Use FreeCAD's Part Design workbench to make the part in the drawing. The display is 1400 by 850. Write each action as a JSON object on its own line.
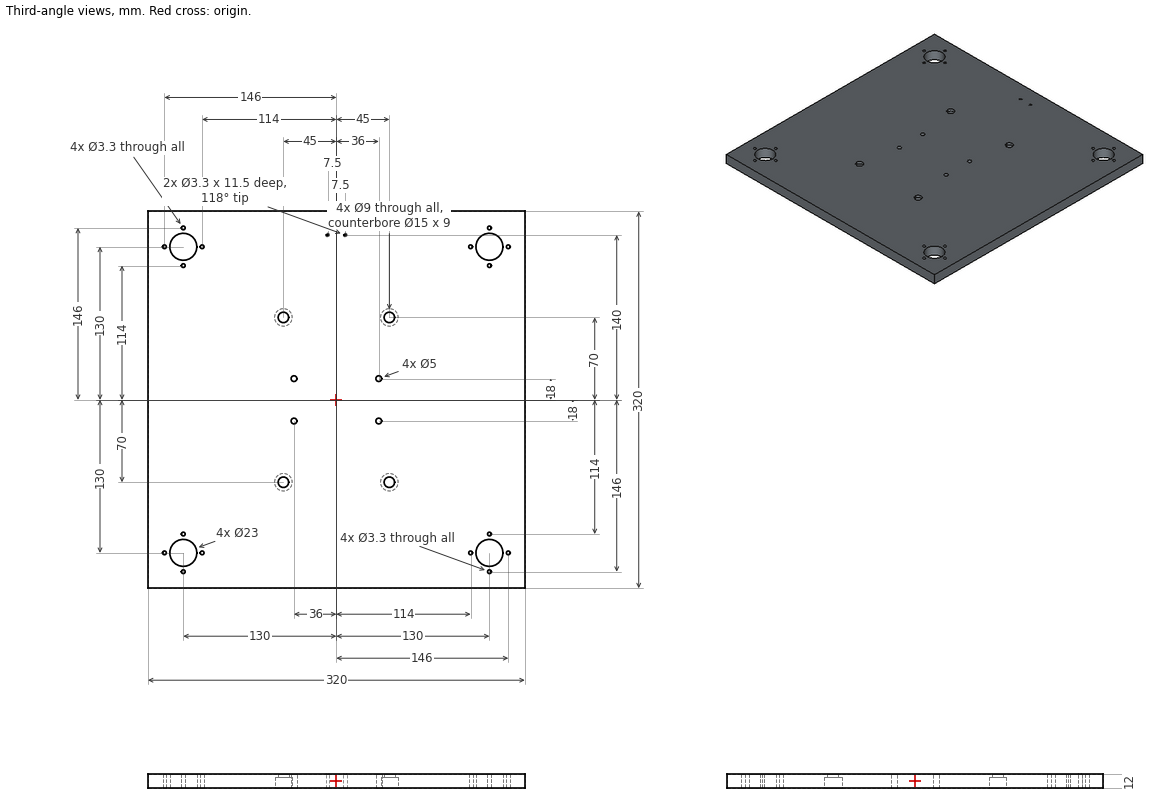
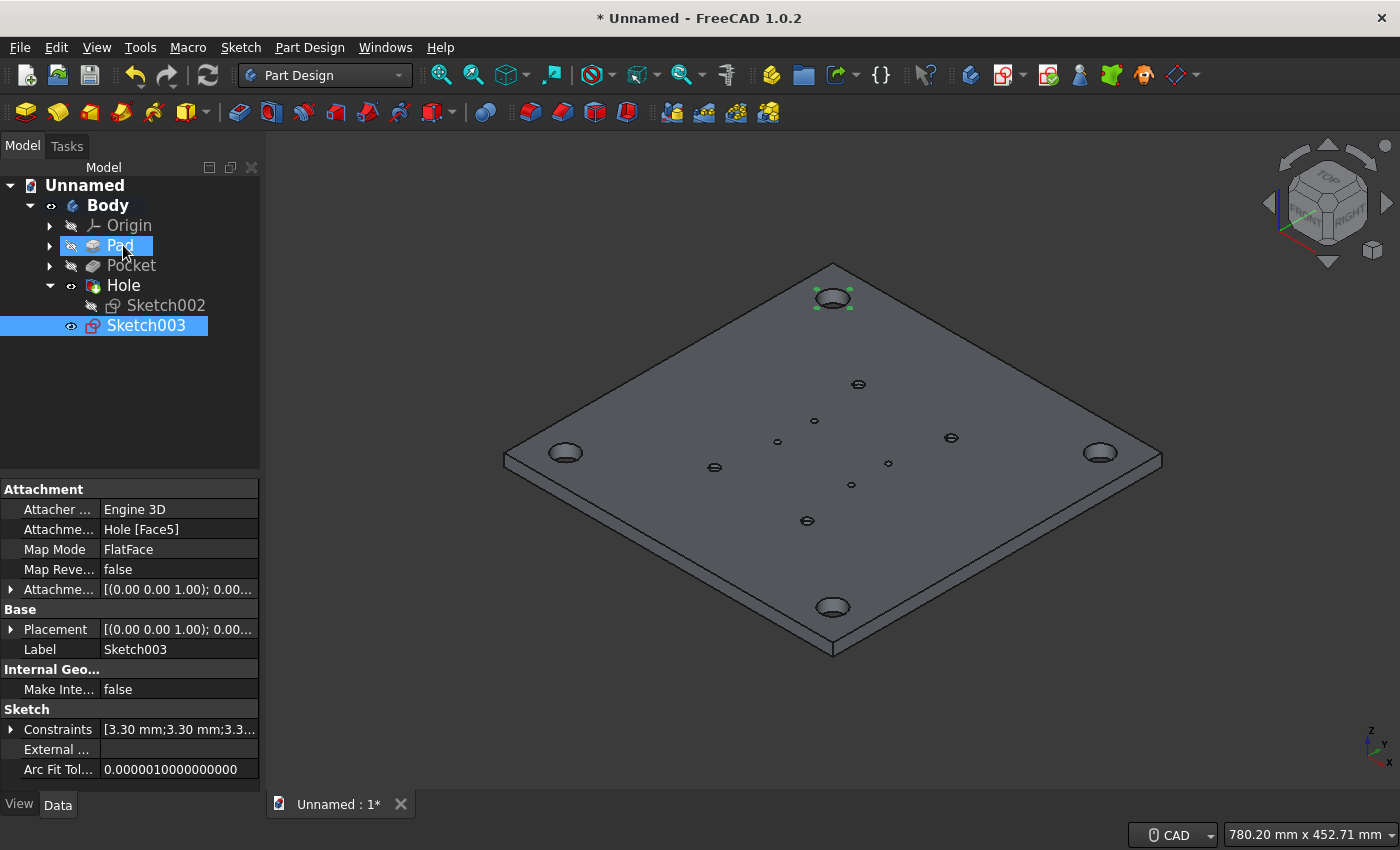
{"action": "left_click", "coordinate": [272, 112]}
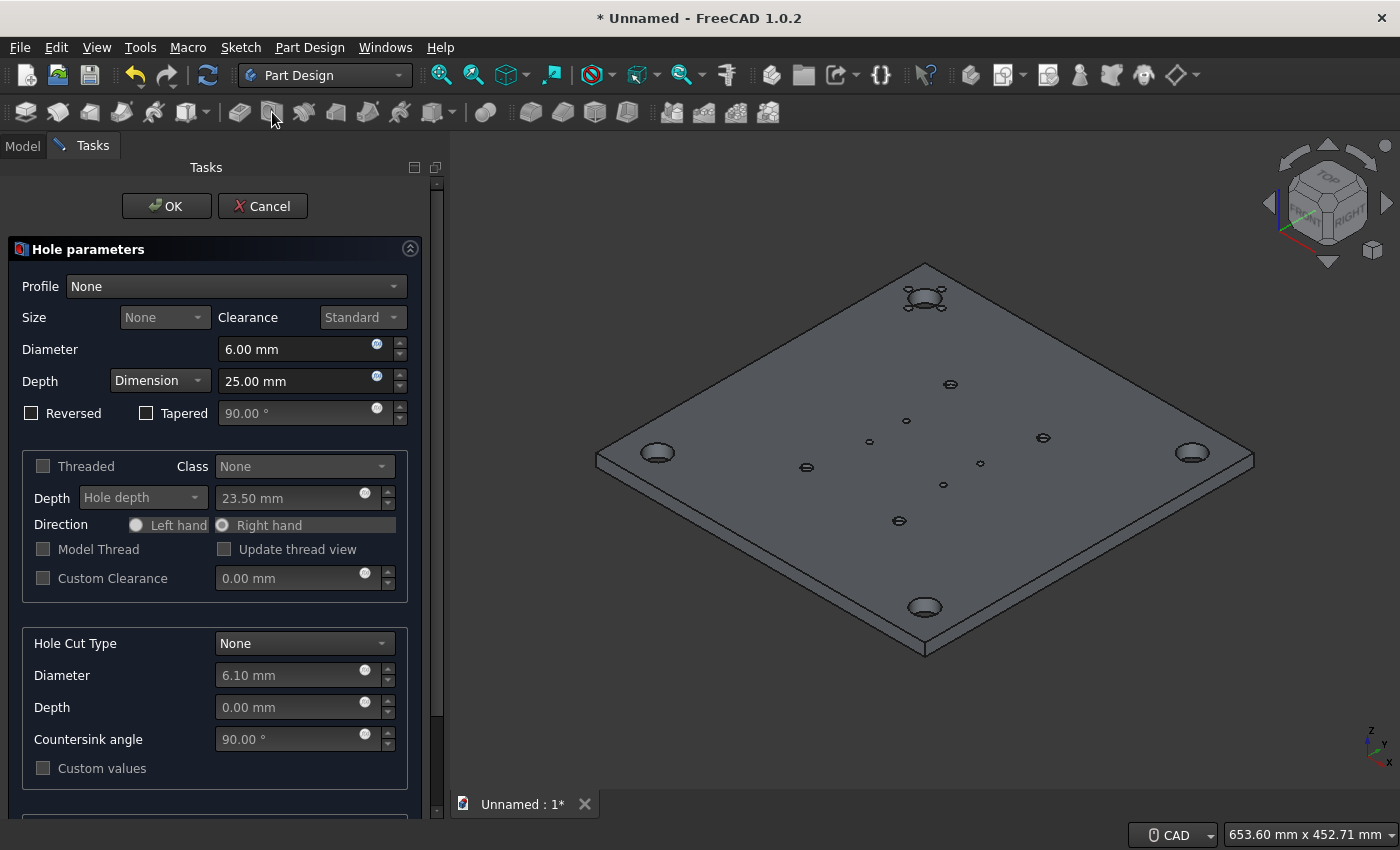
{"action": "triple_click", "coordinate": [305, 349]}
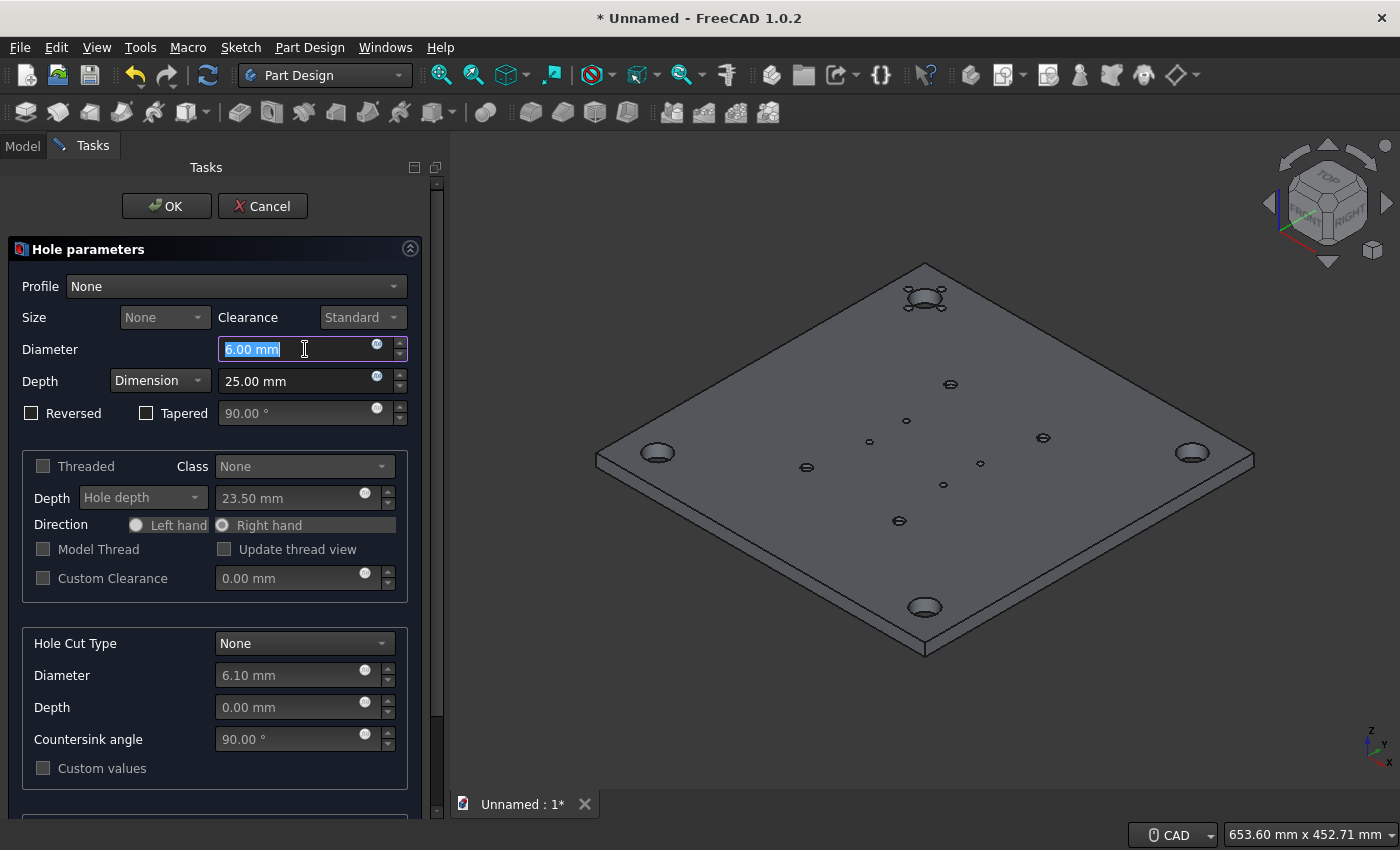
{"action": "type", "text": "3.3"}
{"action": "key", "text": "Tab"}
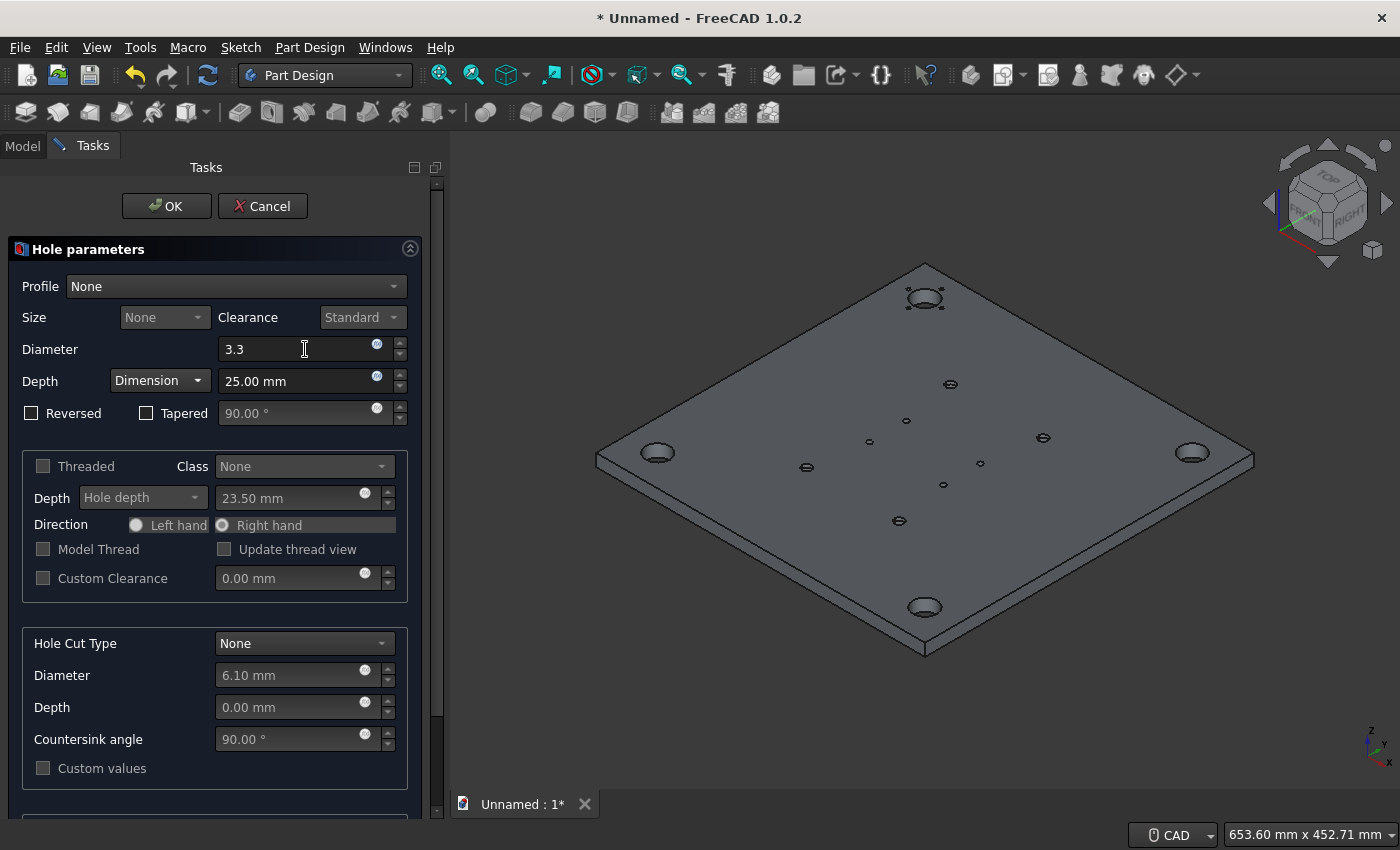
{"action": "left_click", "coordinate": [161, 380]}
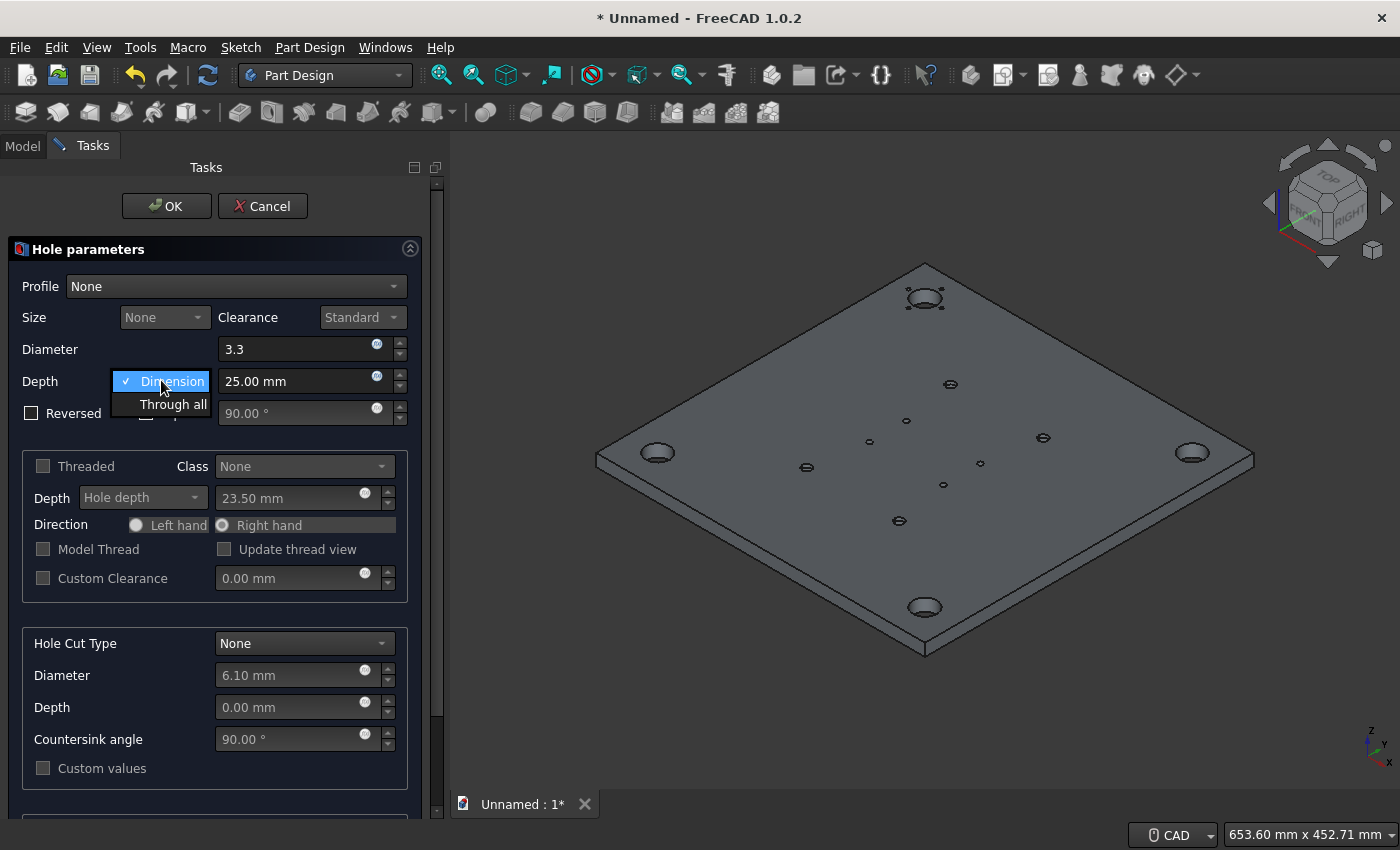
{"action": "left_click", "coordinate": [160, 404]}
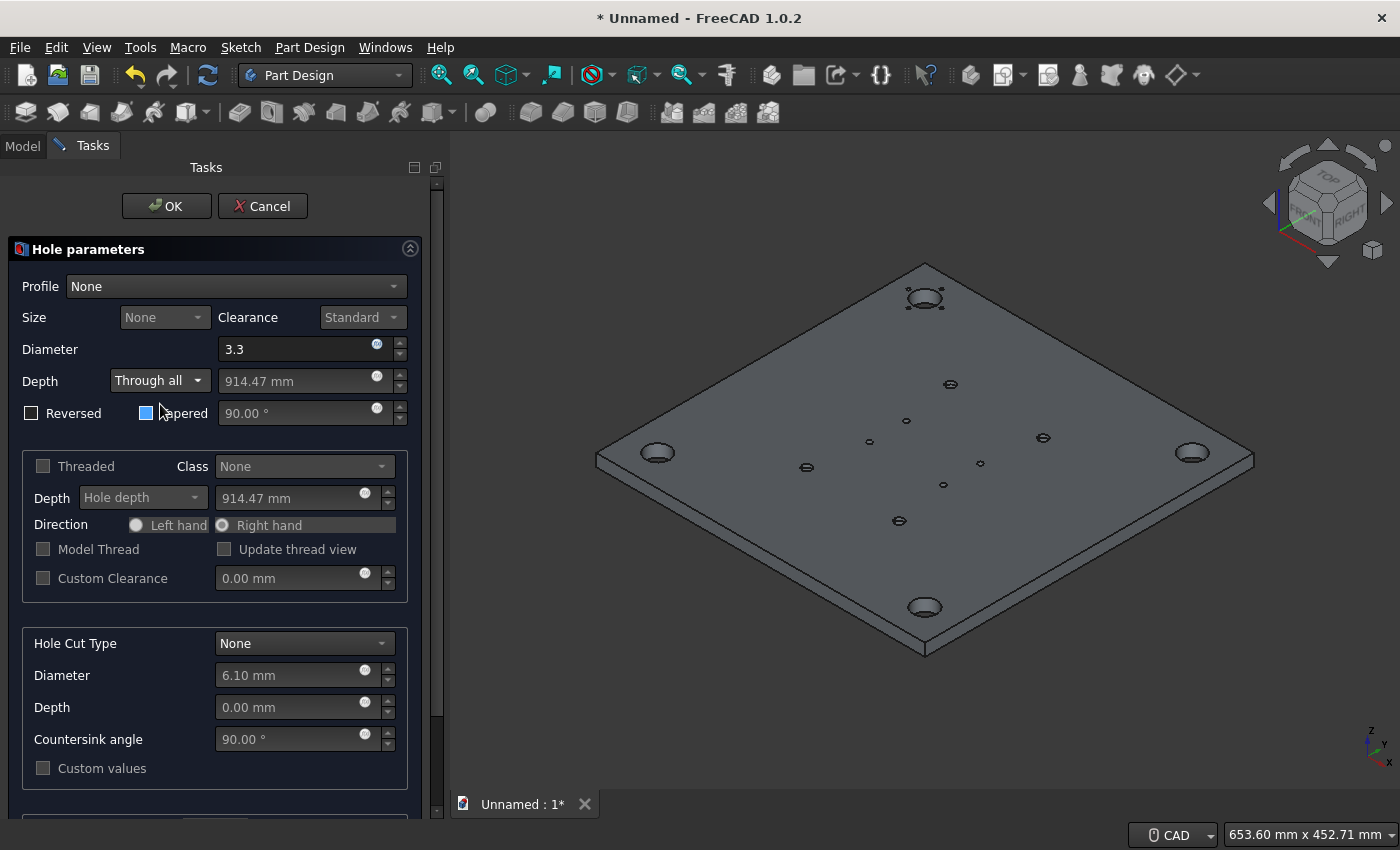
{"action": "left_click", "coordinate": [167, 206]}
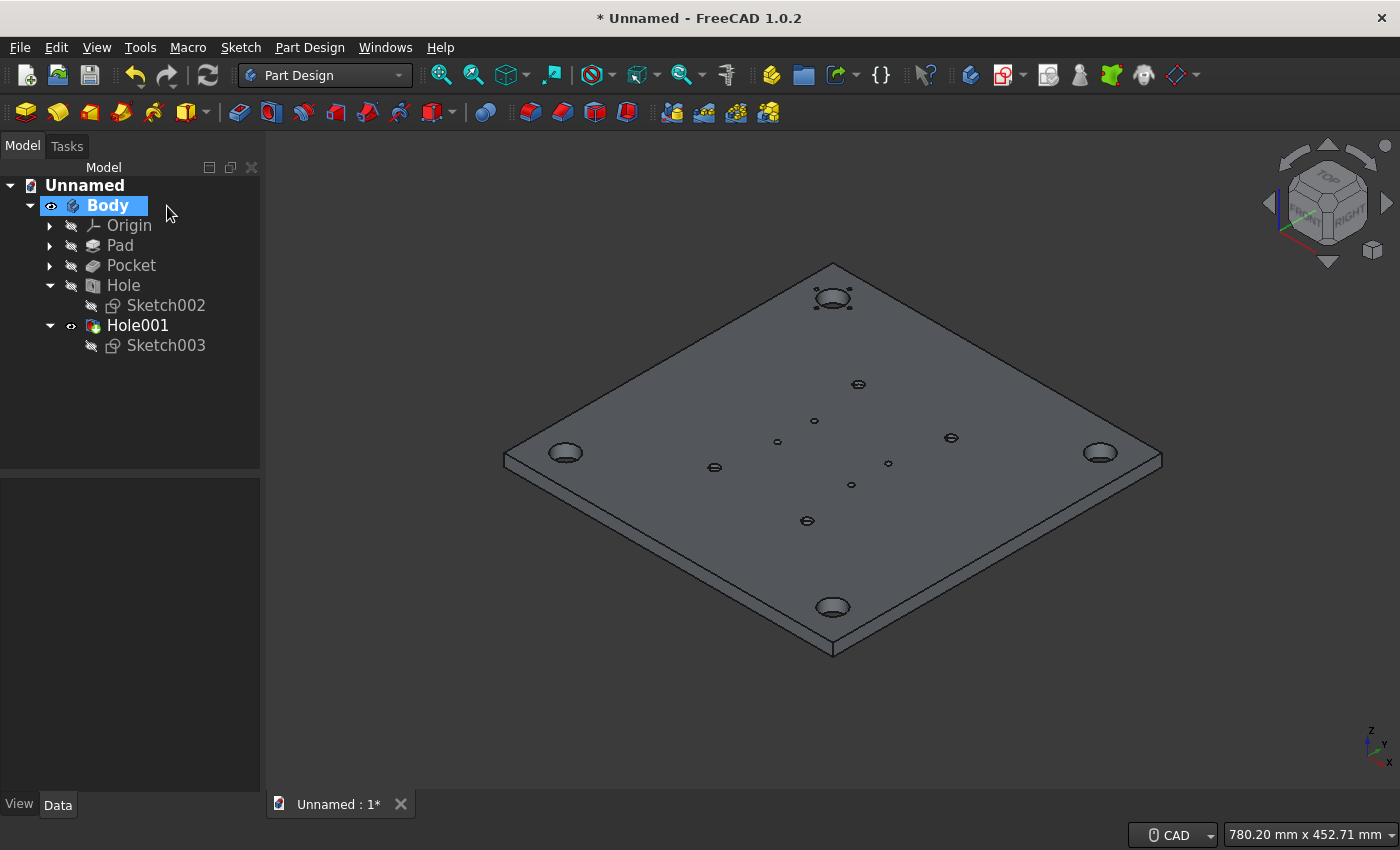
{"action": "left_click", "coordinate": [116, 326]}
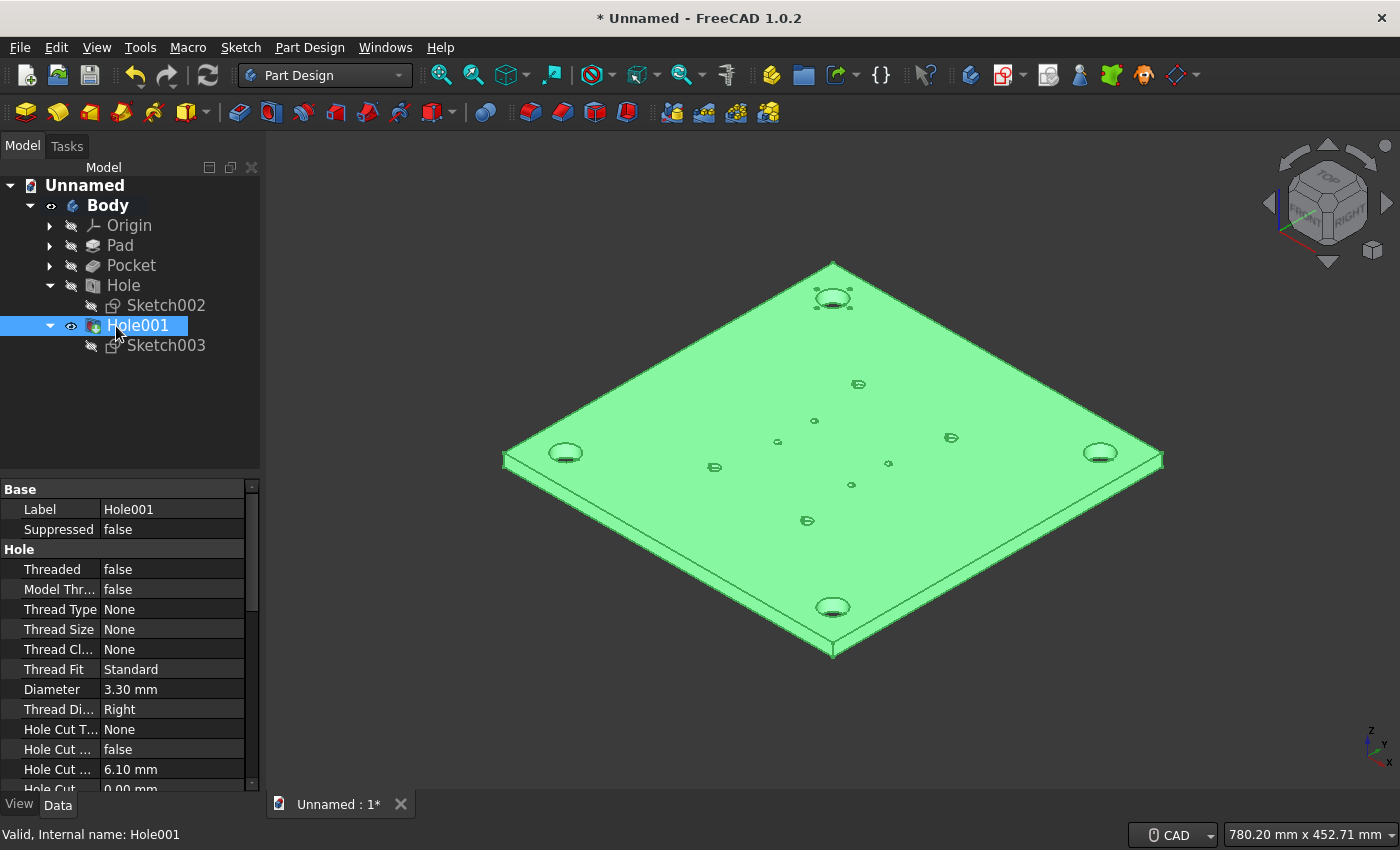
{"action": "left_click", "coordinate": [672, 112]}